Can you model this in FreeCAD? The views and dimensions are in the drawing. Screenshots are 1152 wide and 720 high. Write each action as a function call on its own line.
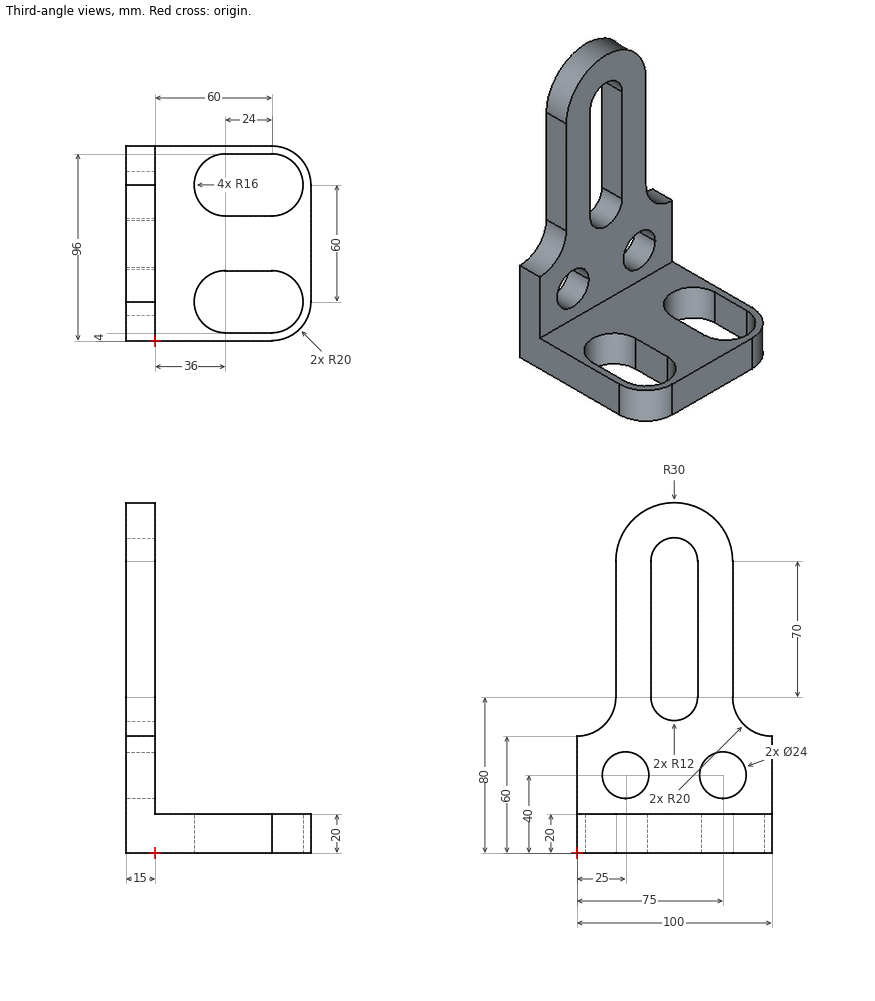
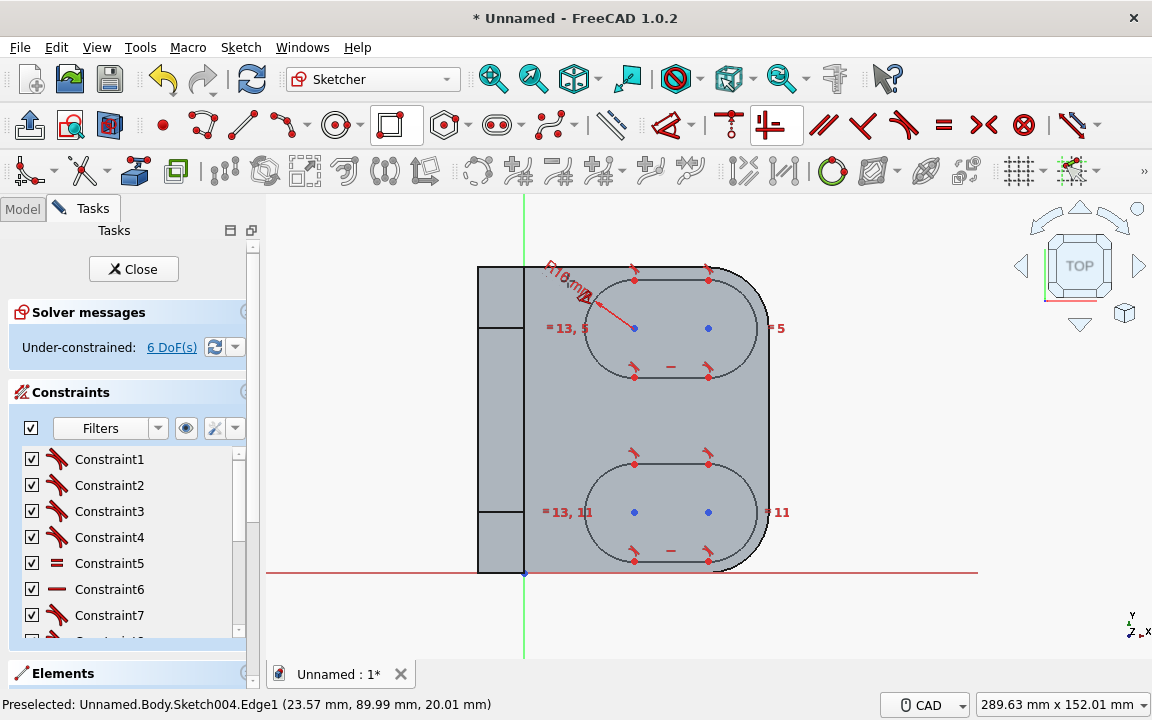
click(656, 280)
click(671, 246)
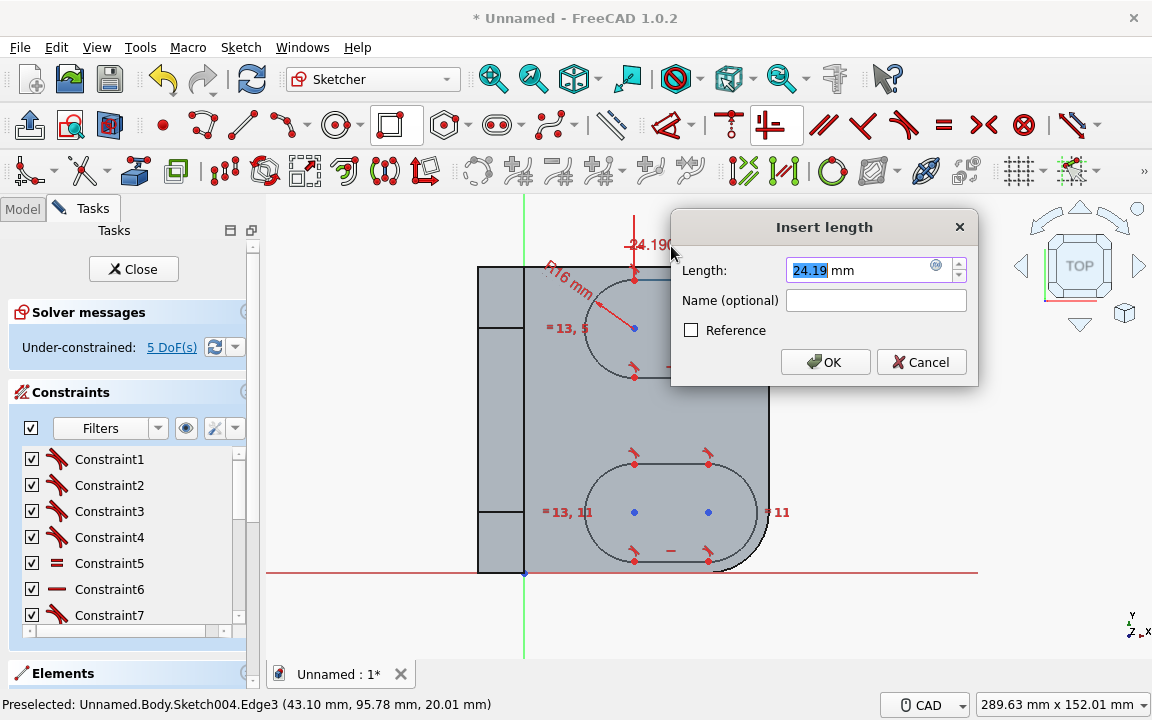
text(24)
key(Return)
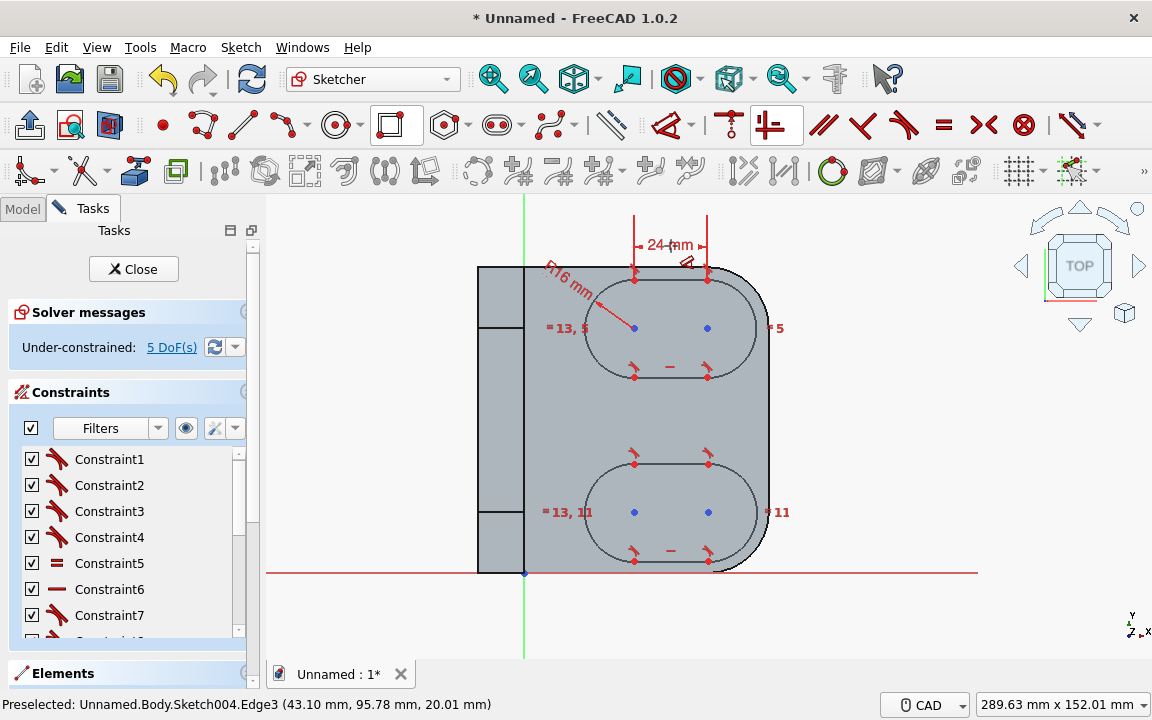
click(656, 464)
click(671, 498)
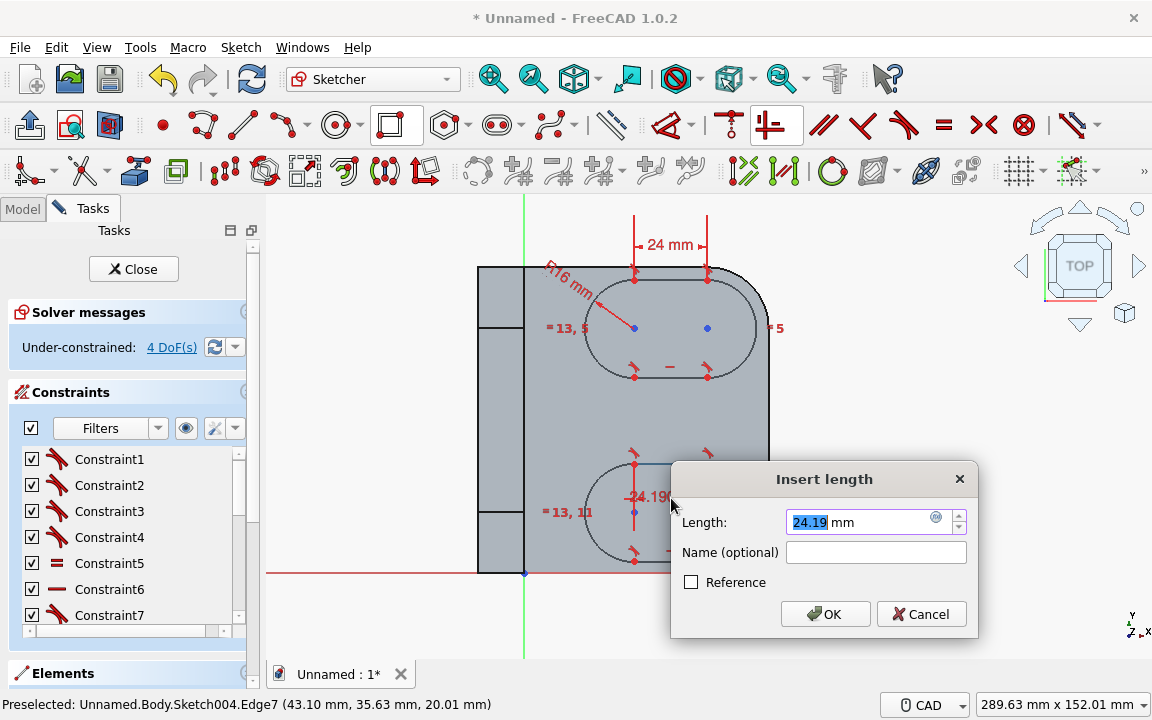
text(24)
key(Return)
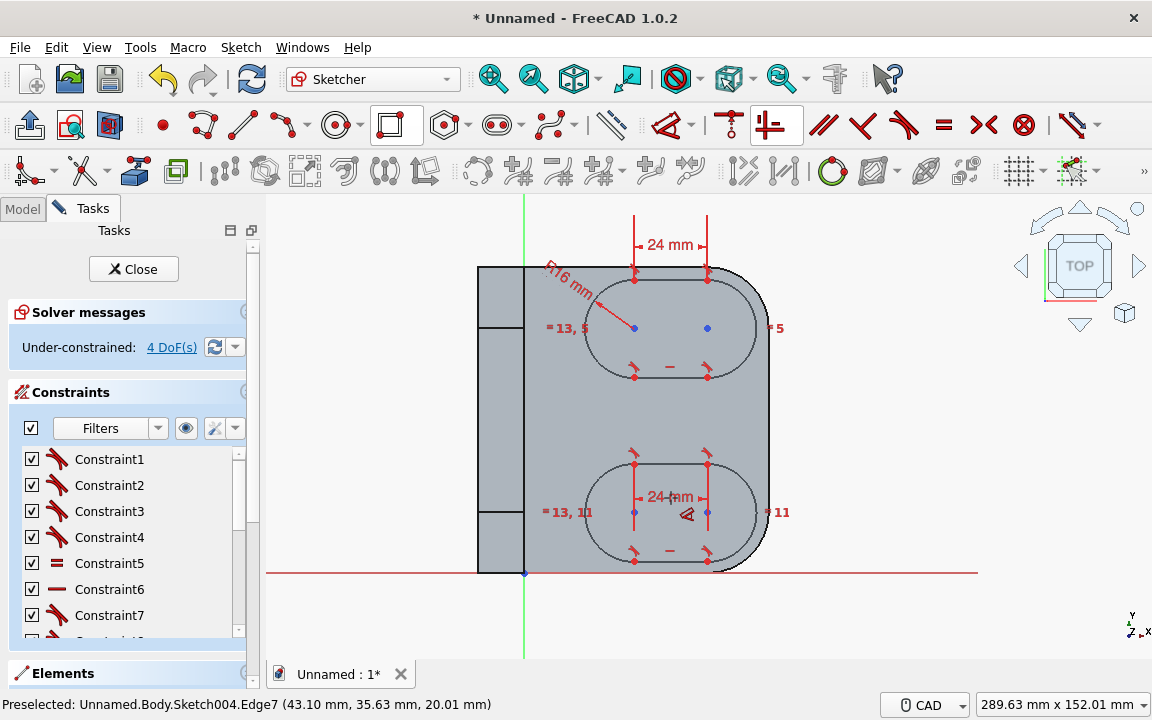
scroll(634, 562, up, 6)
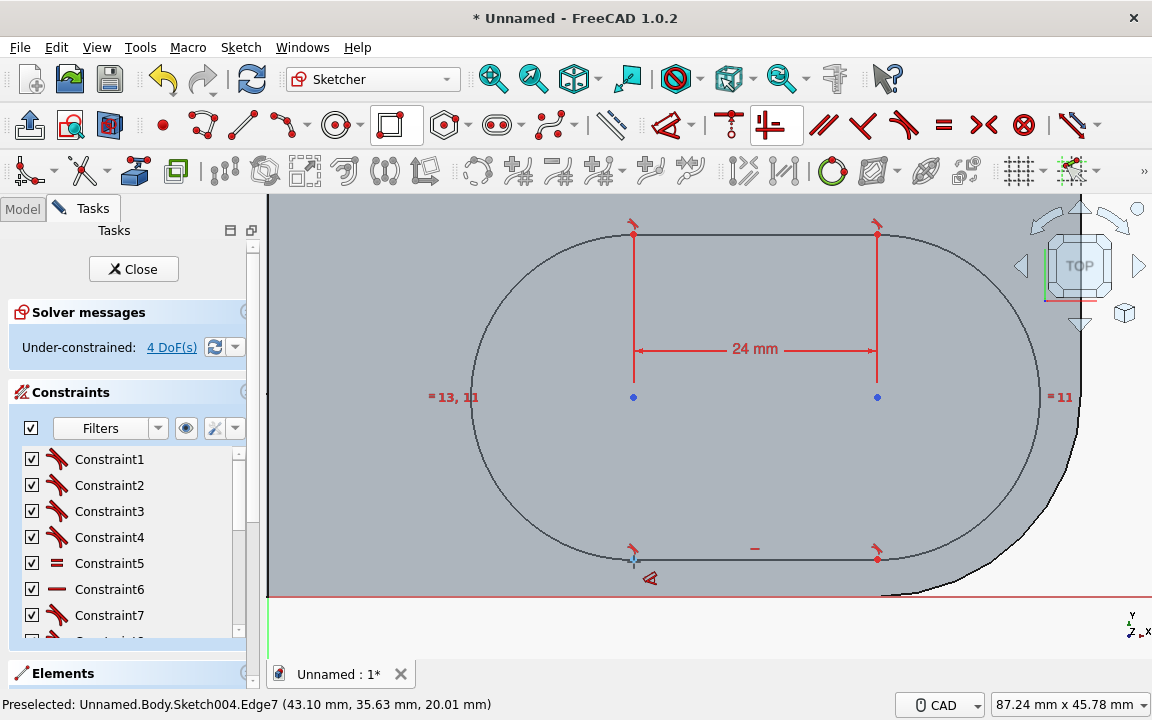
click(634, 560)
click(668, 578)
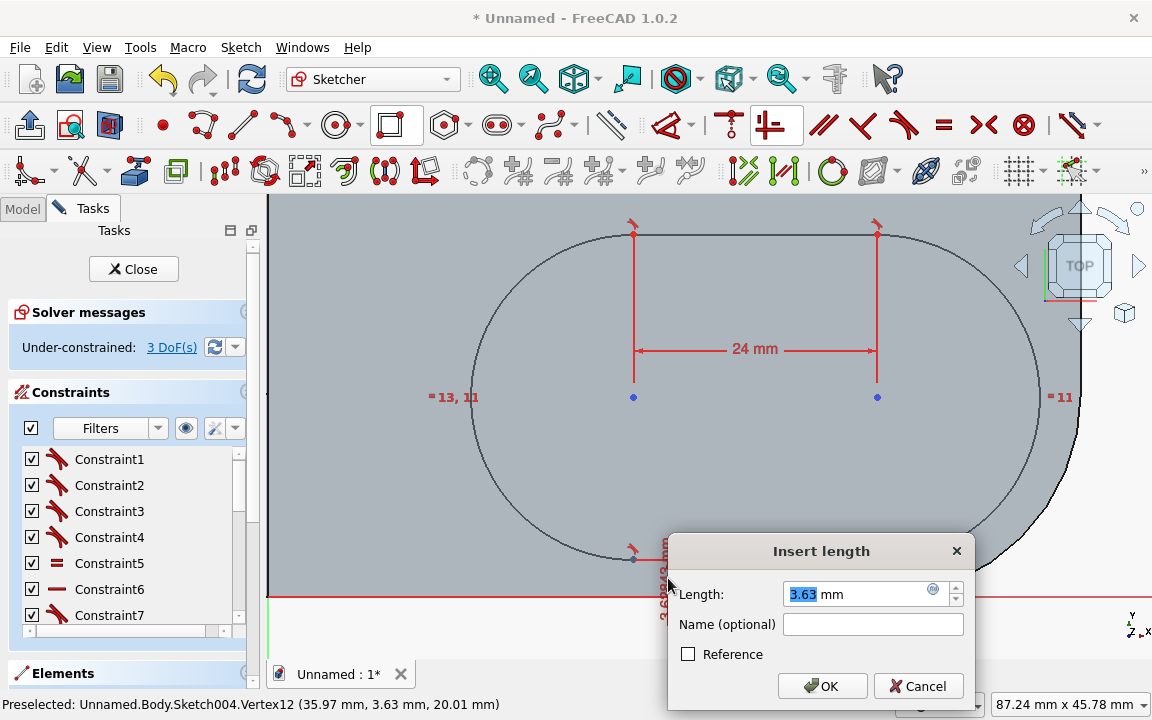
text(4)
key(Return)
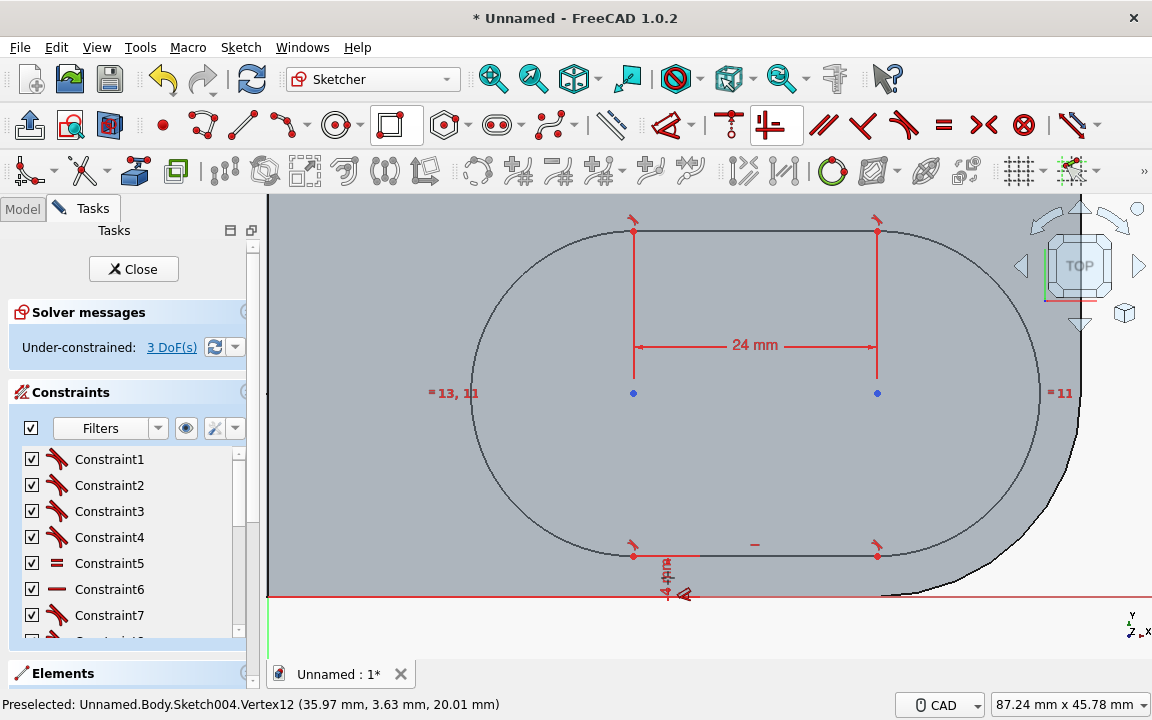
scroll(635, 563, down, 6)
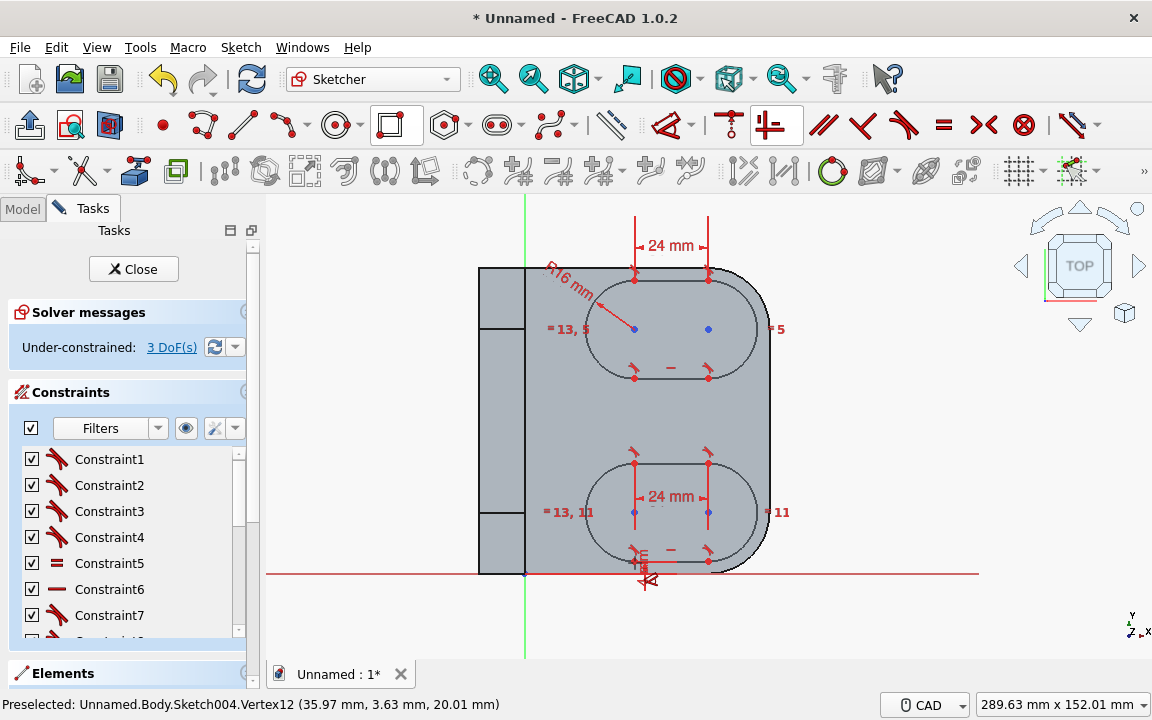
click(635, 281)
click(580, 608)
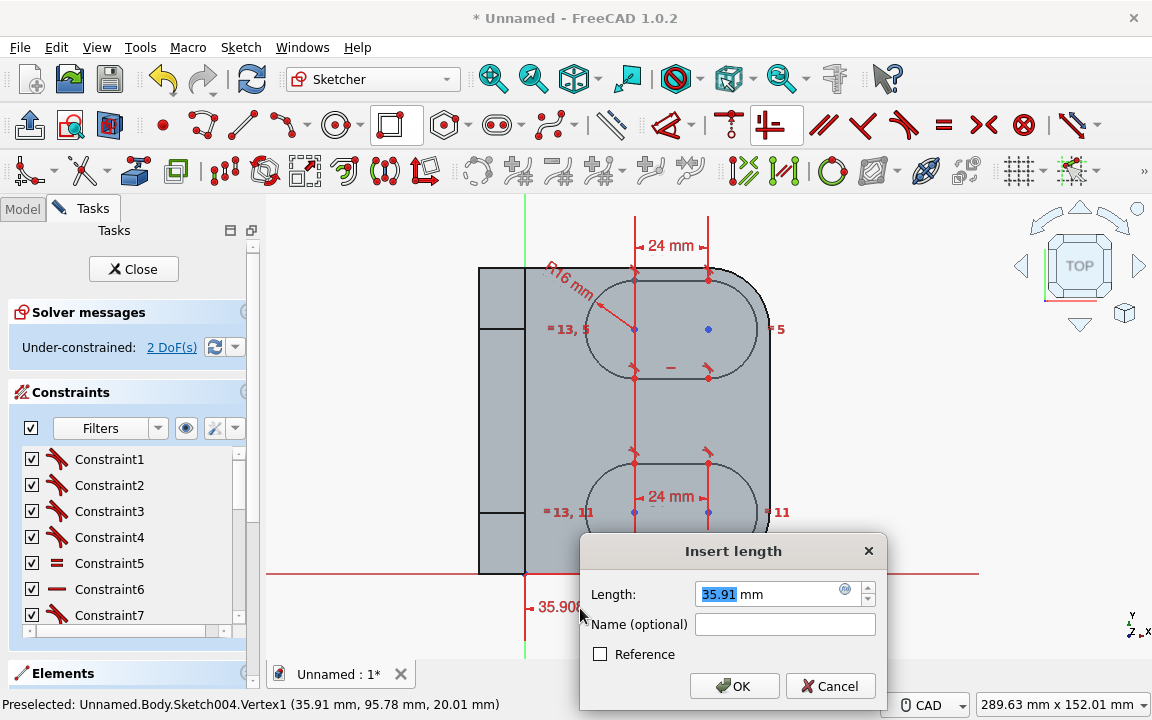
text(36)
key(Return)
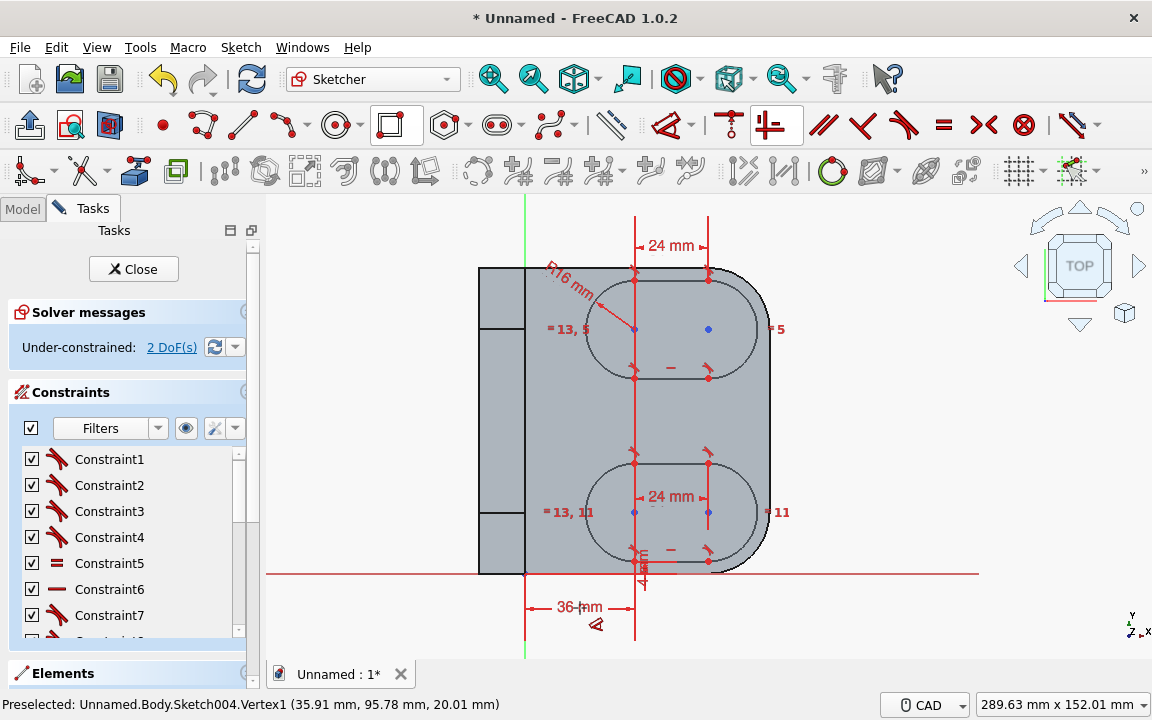
click(635, 281)
click(491, 427)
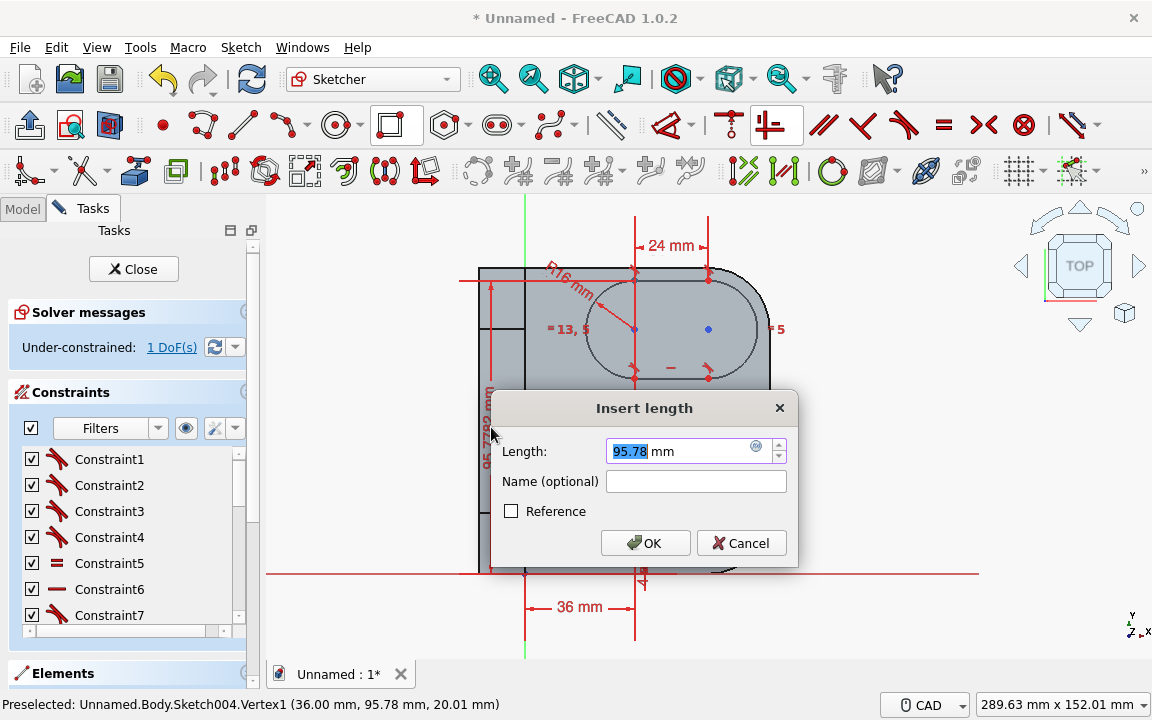
text(96)
key(Return)